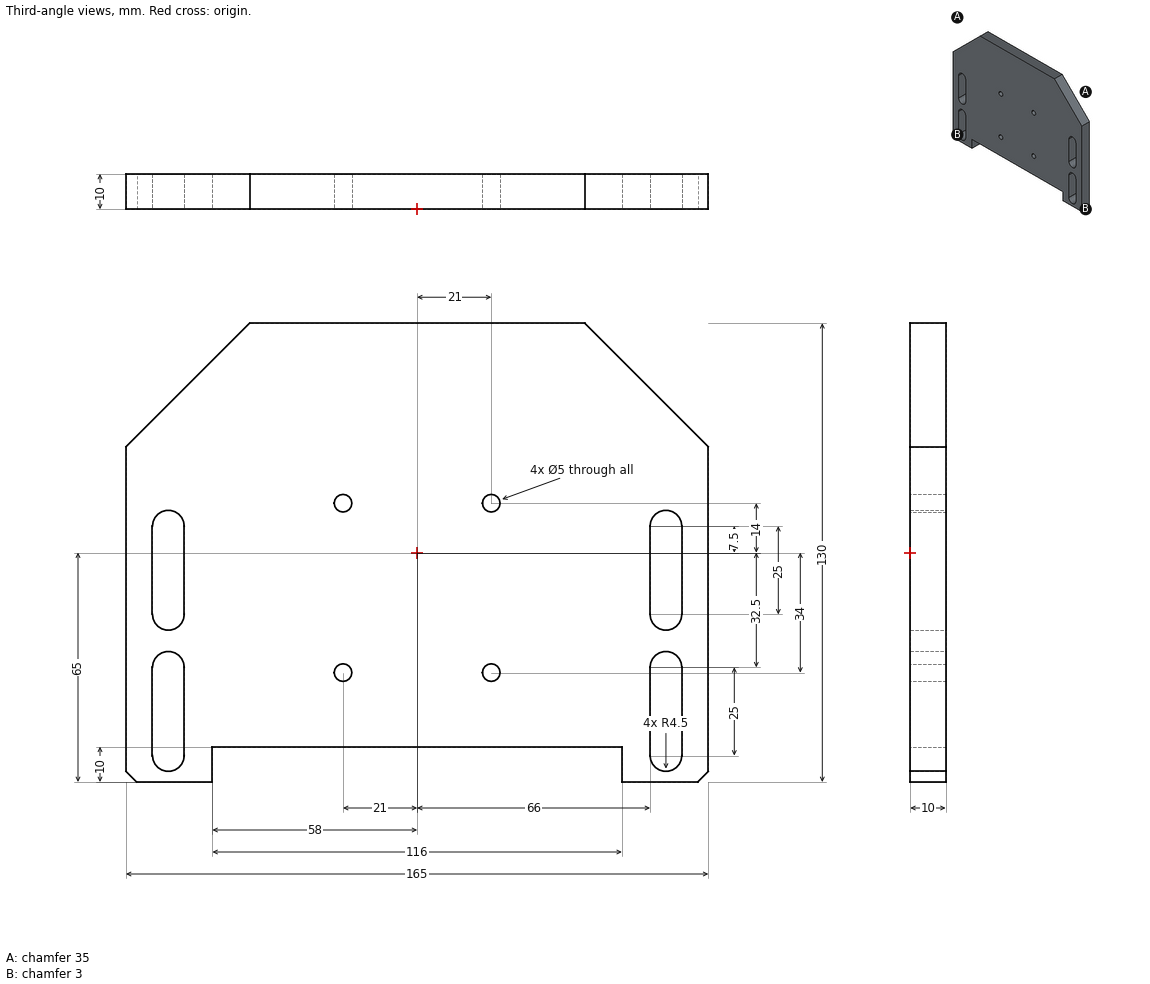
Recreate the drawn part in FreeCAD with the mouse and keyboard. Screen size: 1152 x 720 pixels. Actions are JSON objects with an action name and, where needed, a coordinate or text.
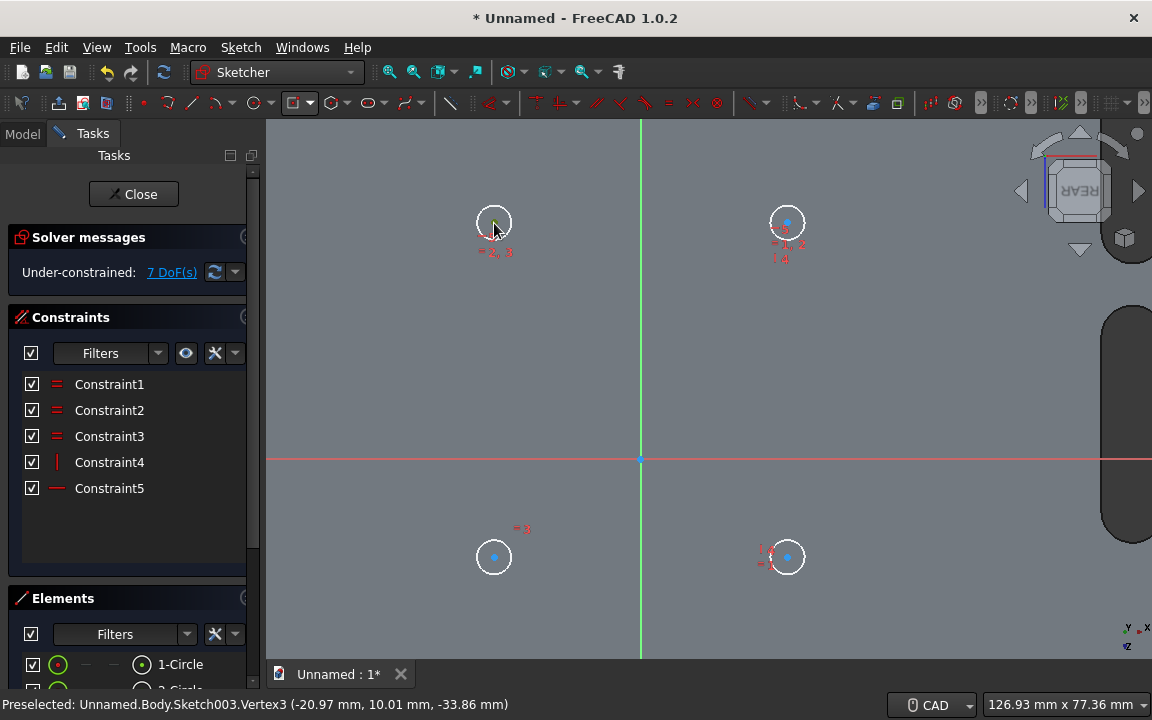
{"action": "left_click", "coordinate": [494, 557]}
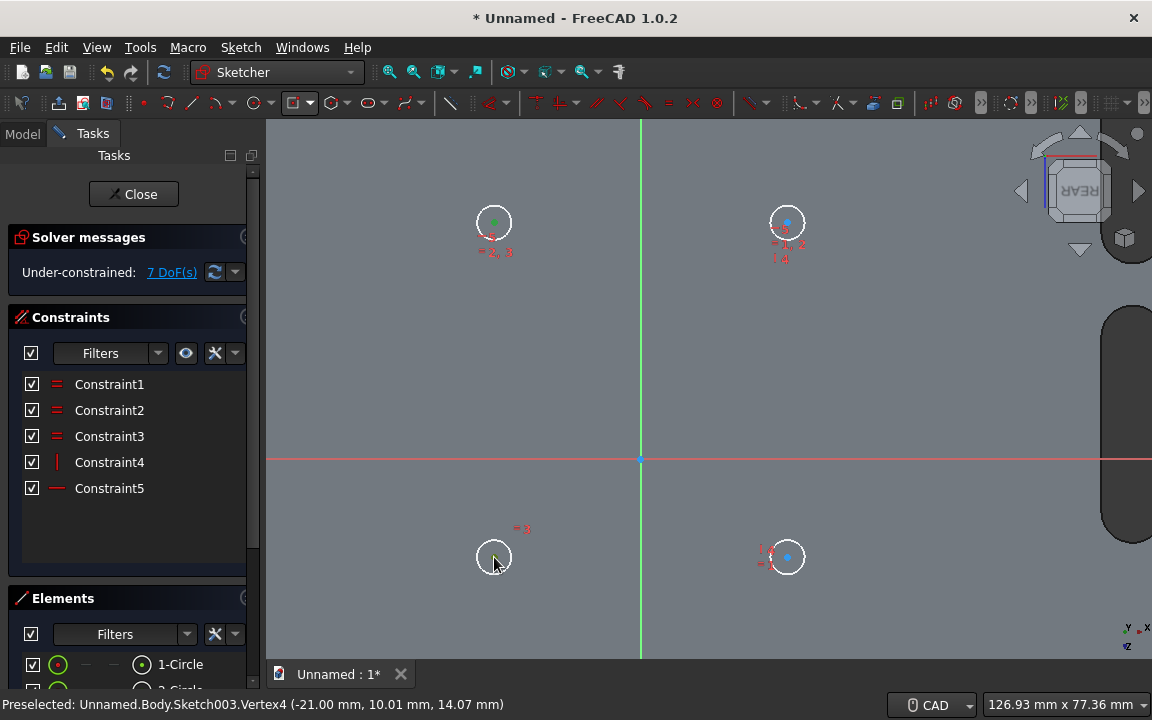
{"action": "key", "text": "v"}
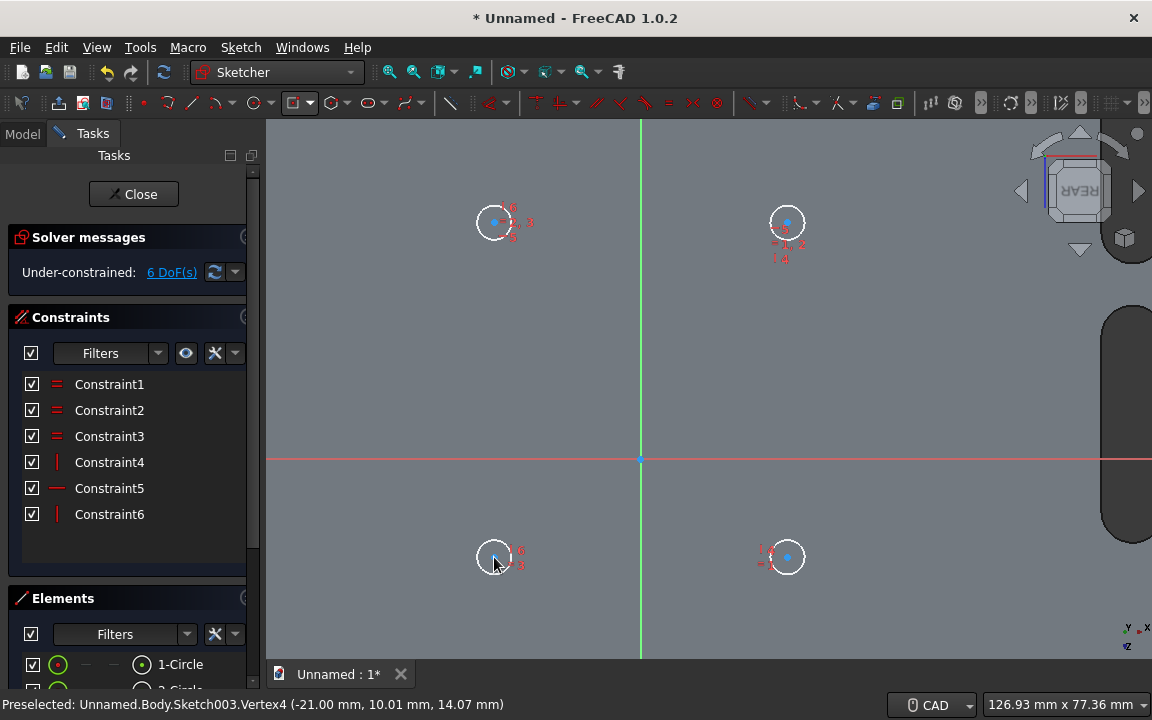
{"action": "left_click", "coordinate": [788, 557]}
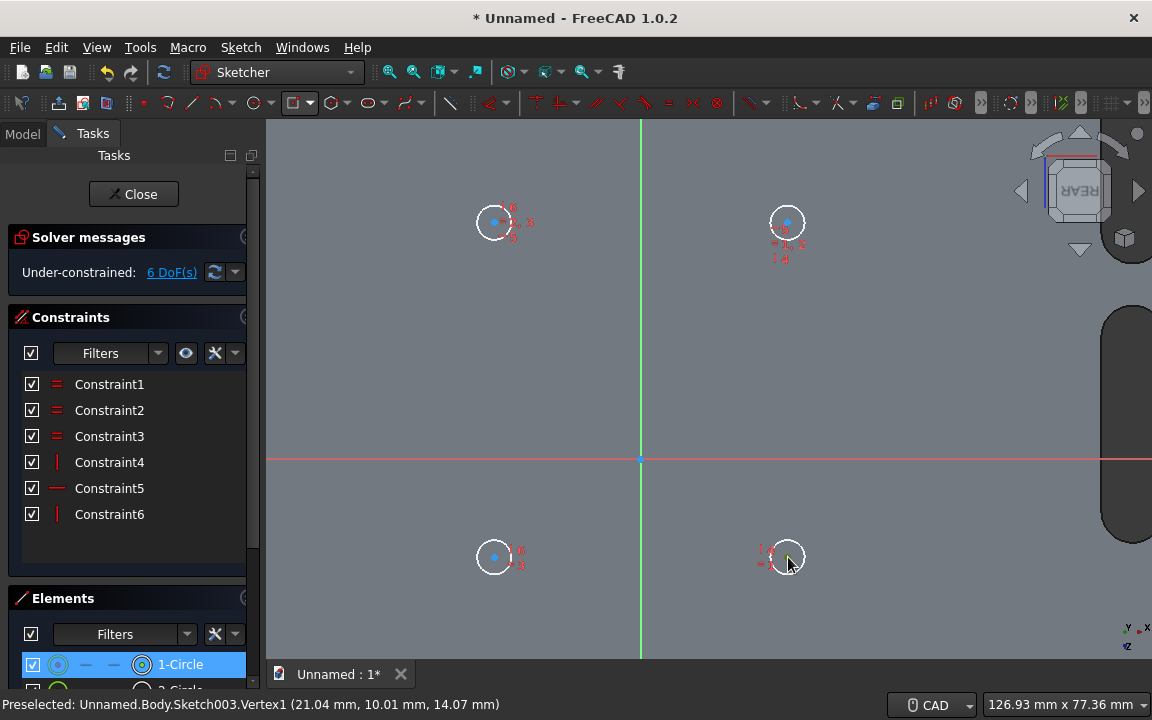
{"action": "left_click", "coordinate": [494, 557]}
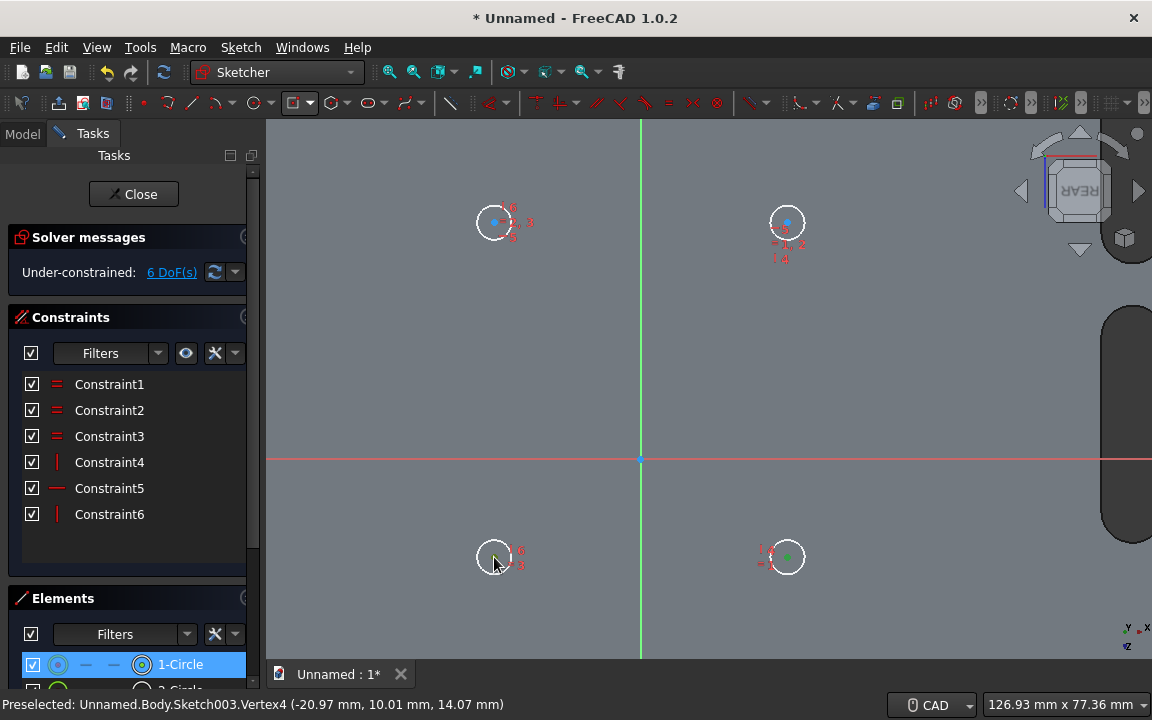
{"action": "key", "text": "h"}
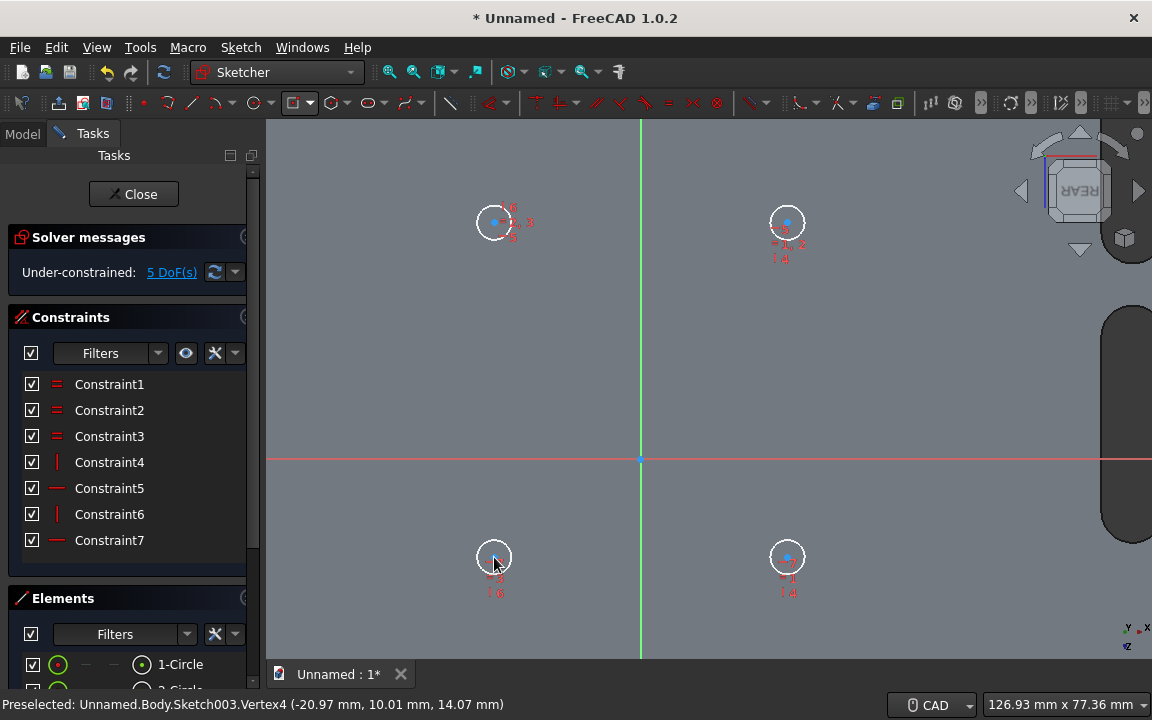
{"action": "left_click", "coordinate": [490, 104]}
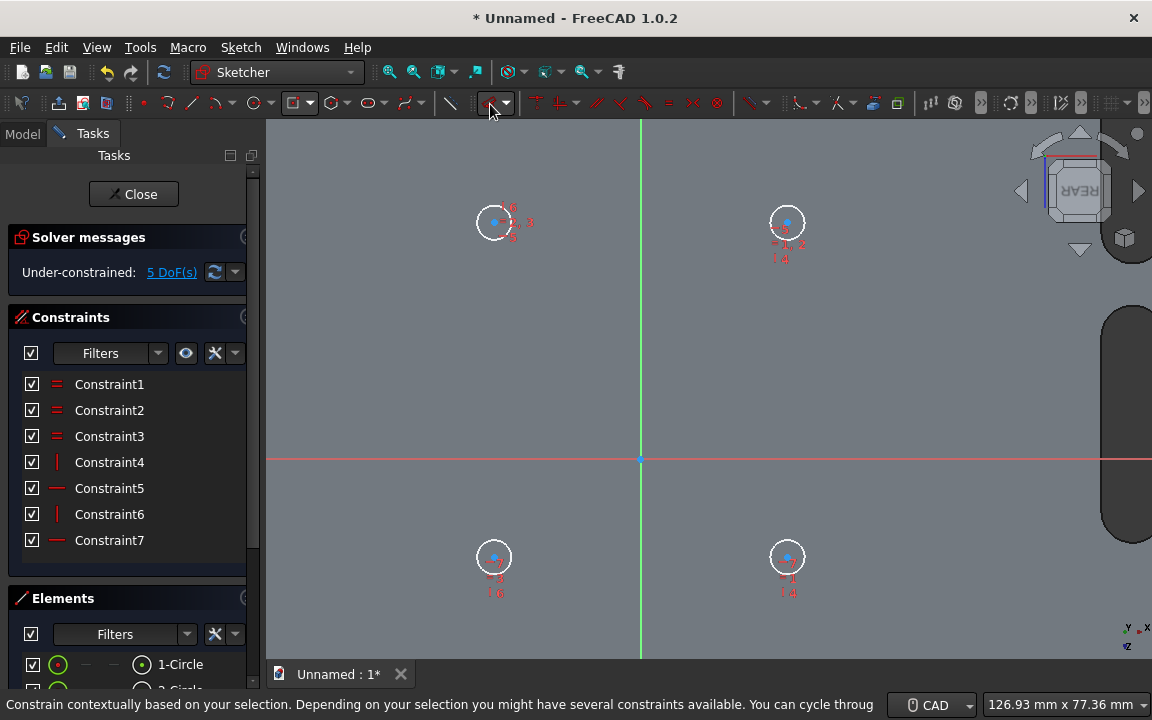
{"action": "left_click", "coordinate": [800, 545]}
{"action": "left_click", "coordinate": [823, 523]}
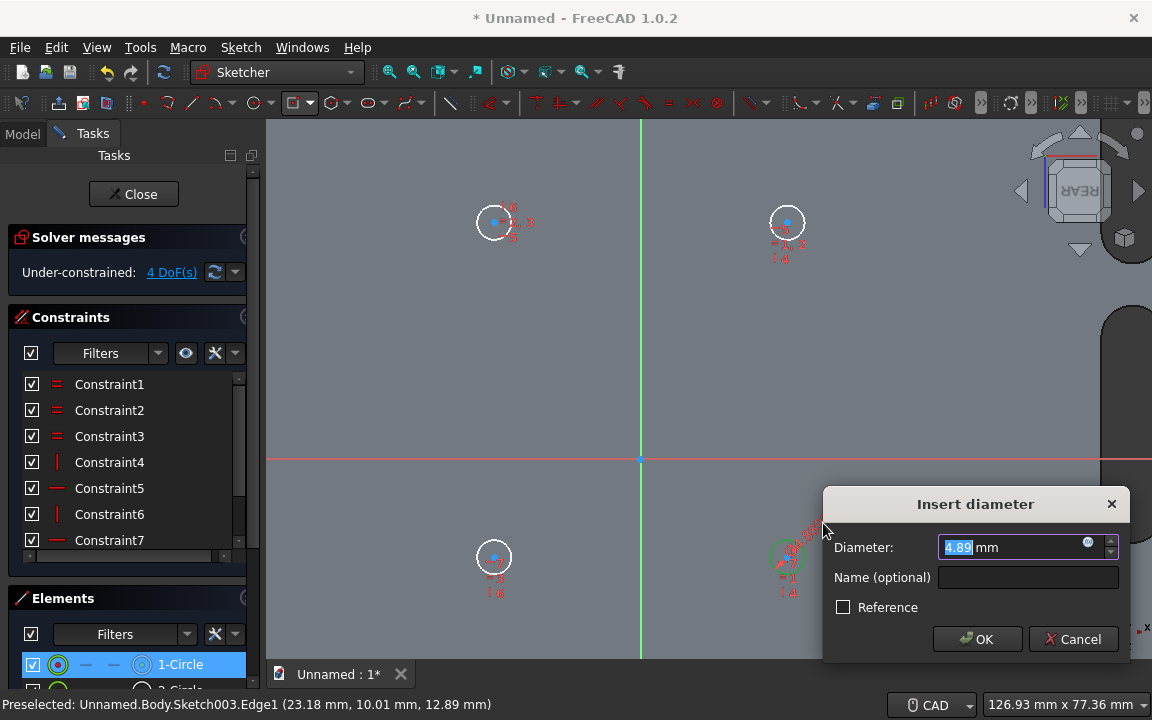
{"action": "type", "text": "5"}
{"action": "key", "text": "Return"}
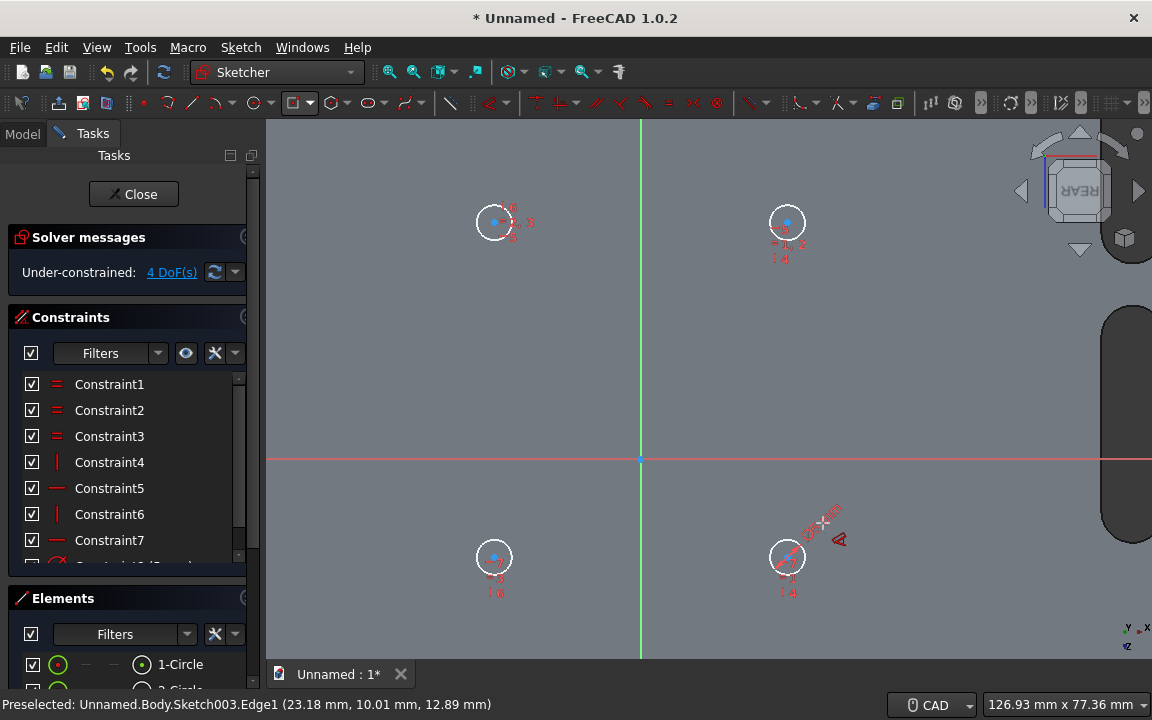
{"action": "left_click", "coordinate": [788, 557]}
{"action": "left_click", "coordinate": [714, 591]}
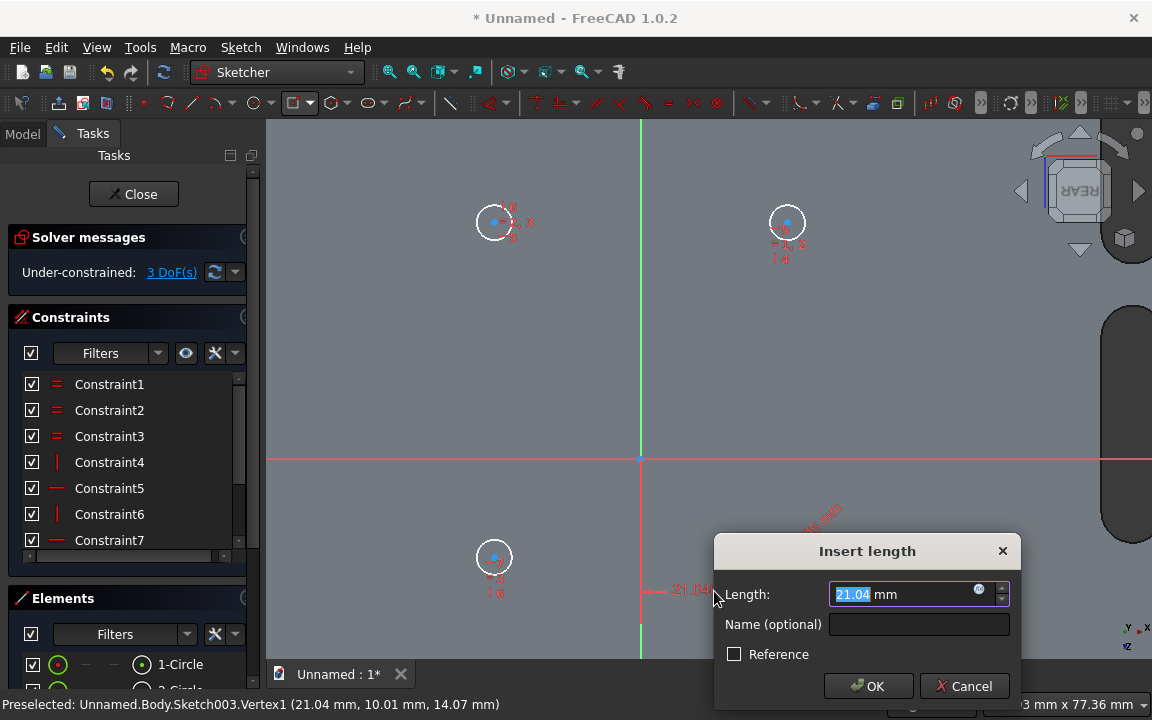
{"action": "type", "text": "21"}
{"action": "key", "text": "Return"}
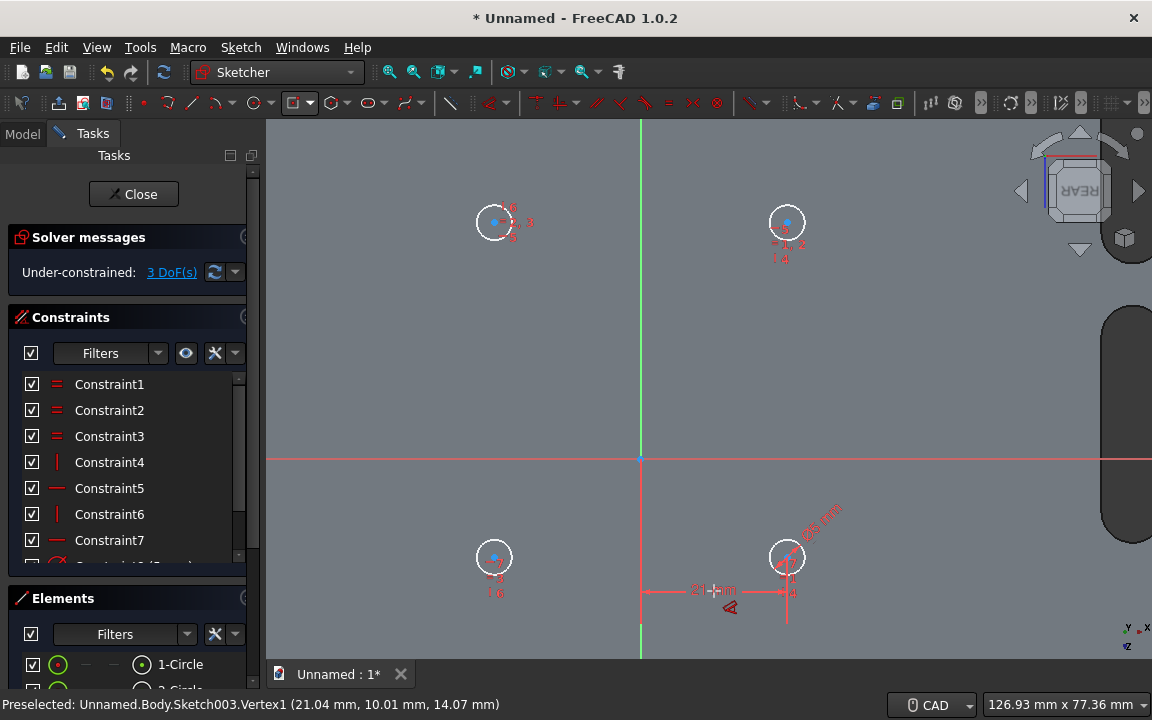
{"action": "left_click", "coordinate": [787, 557]}
{"action": "left_click", "coordinate": [821, 486]}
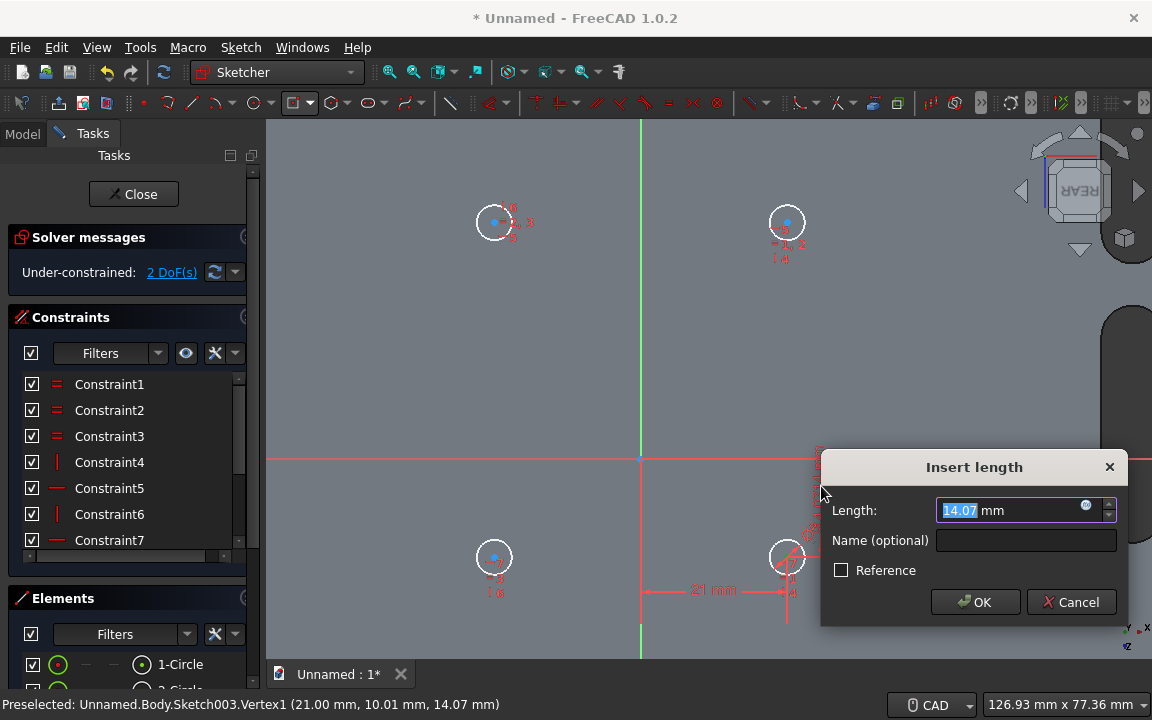
{"action": "type", "text": "14"}
{"action": "key", "text": "Return"}